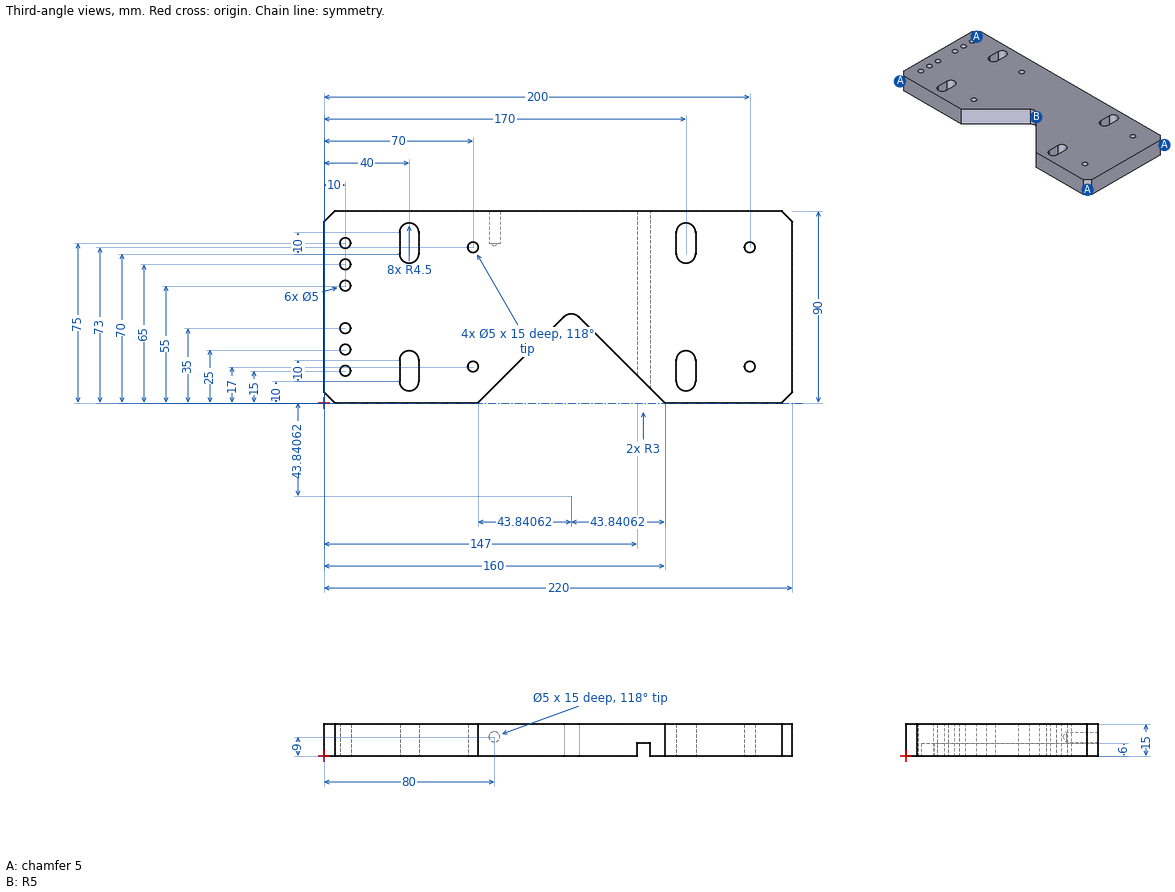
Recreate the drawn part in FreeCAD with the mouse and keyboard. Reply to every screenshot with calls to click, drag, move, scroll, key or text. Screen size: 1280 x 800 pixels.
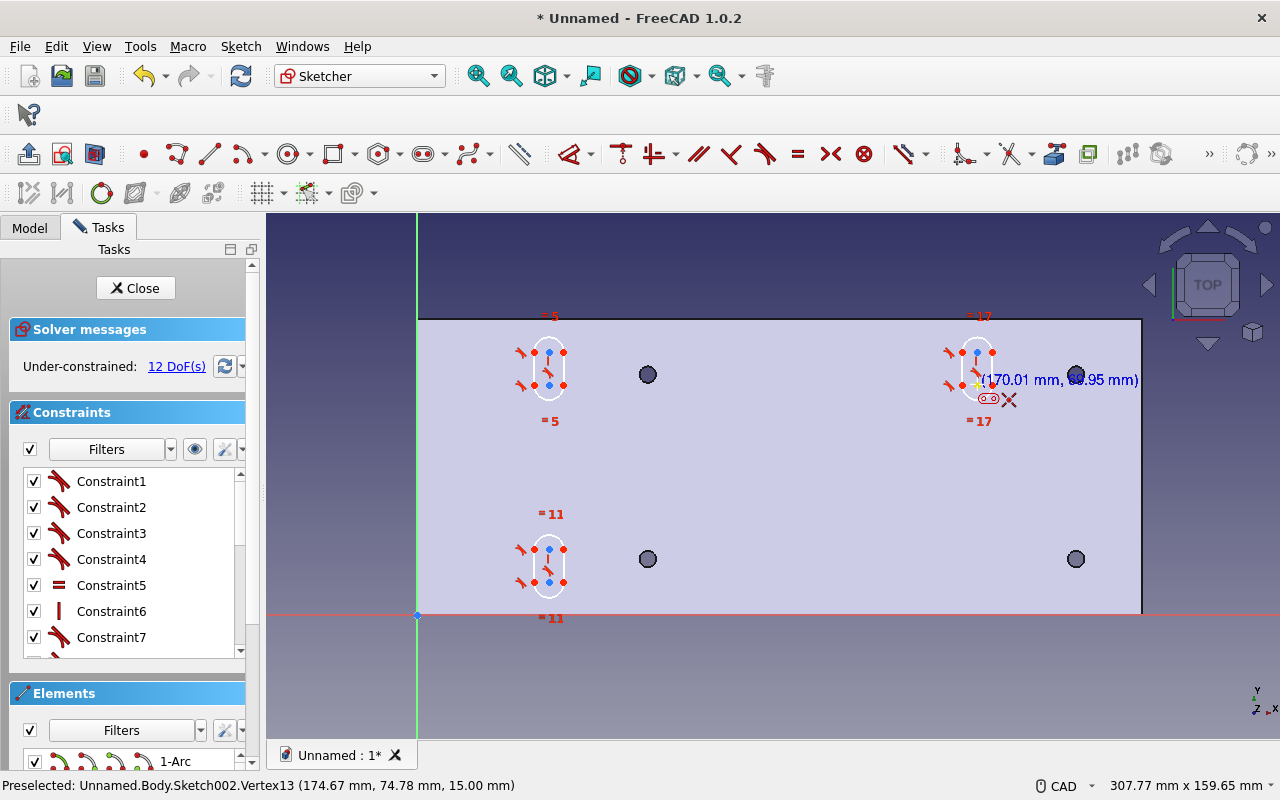
scroll(977, 582, up, 3)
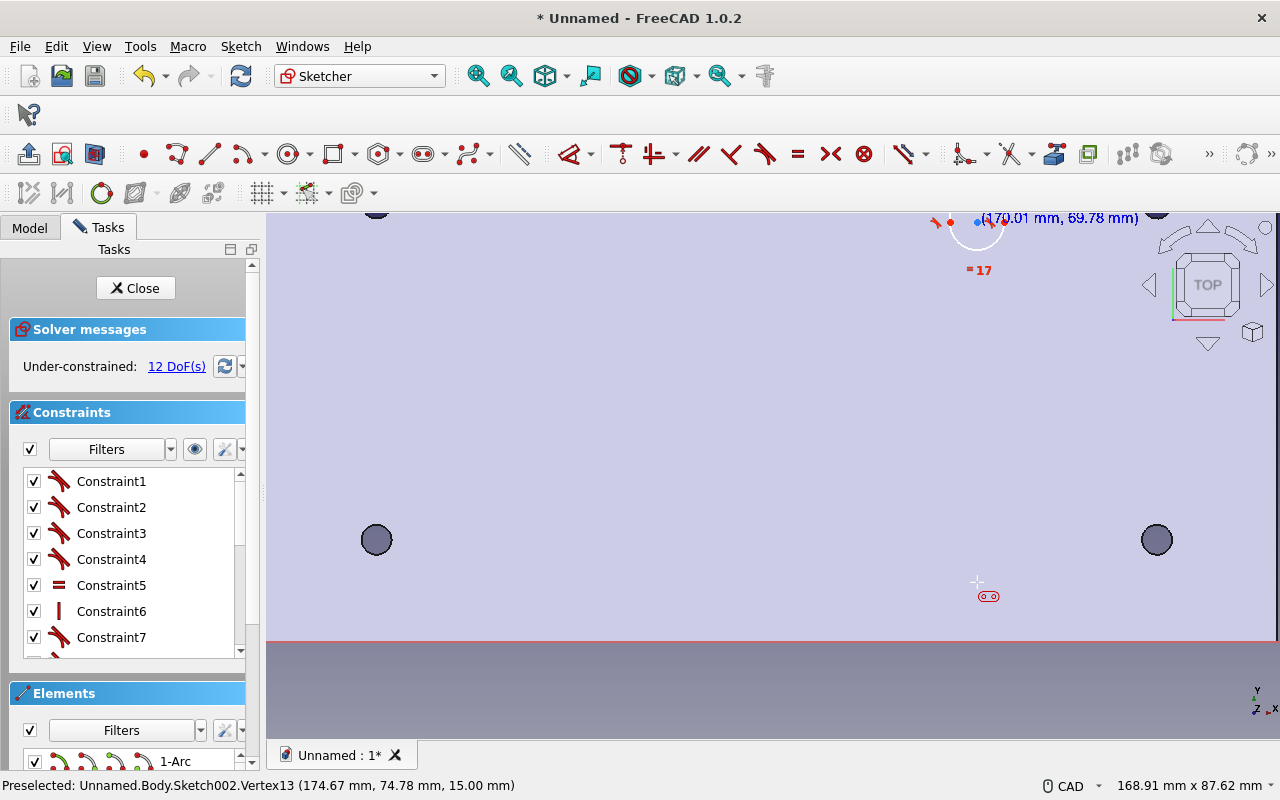
click(977, 582)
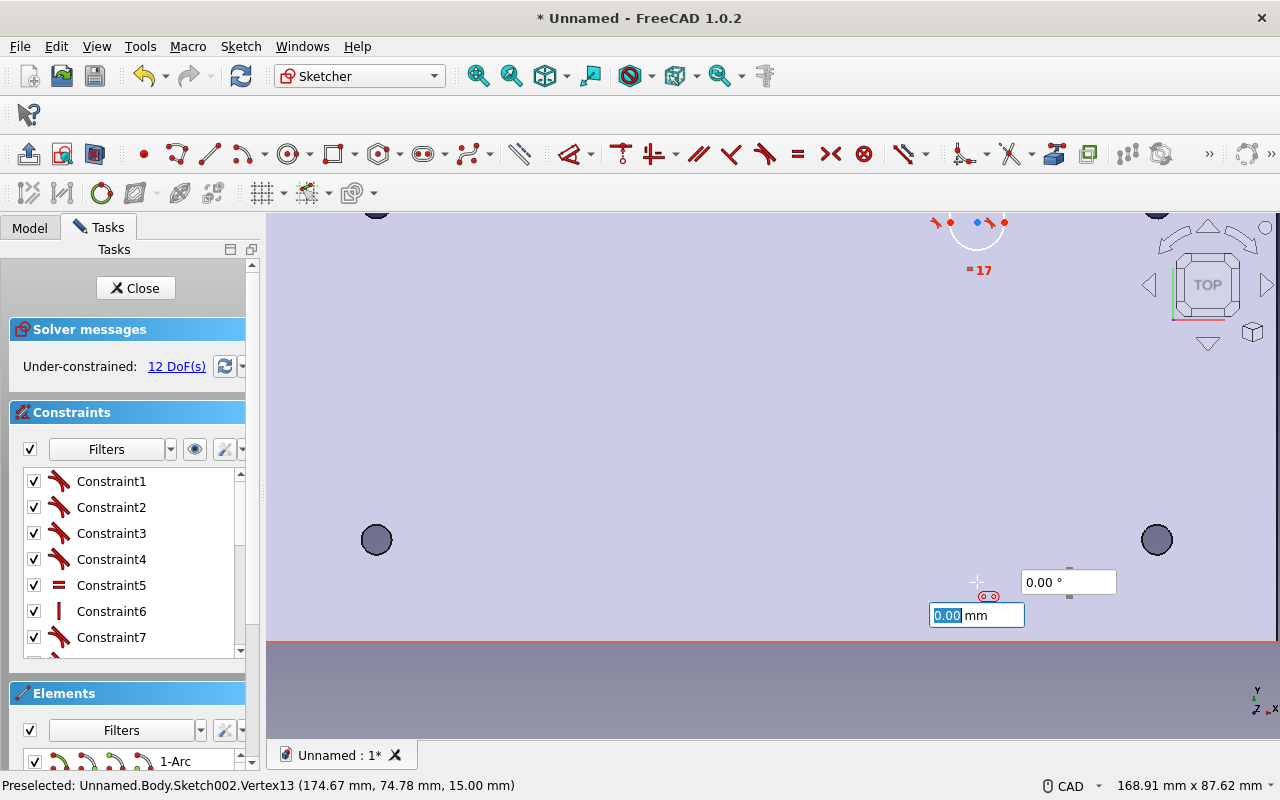
click(977, 522)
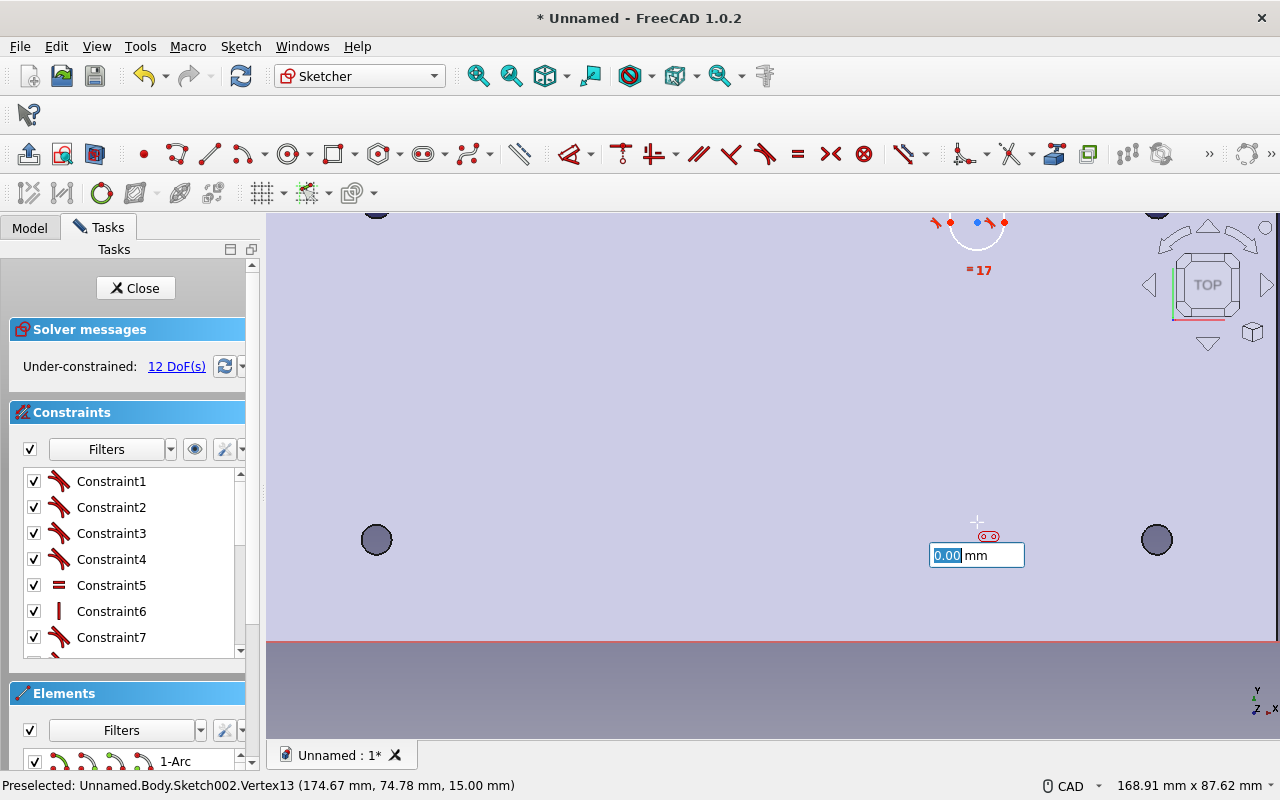
click(1004, 552)
key(Escape)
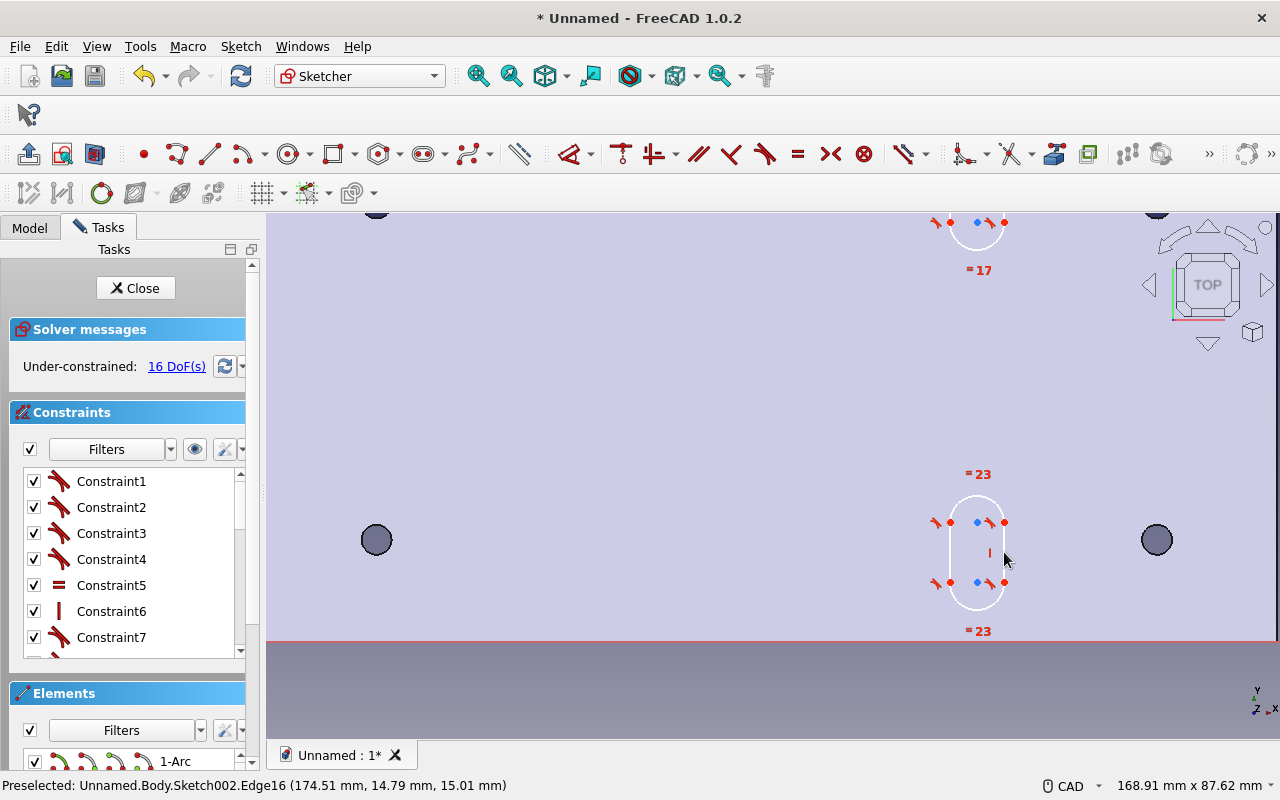
scroll(977, 583, down, 3)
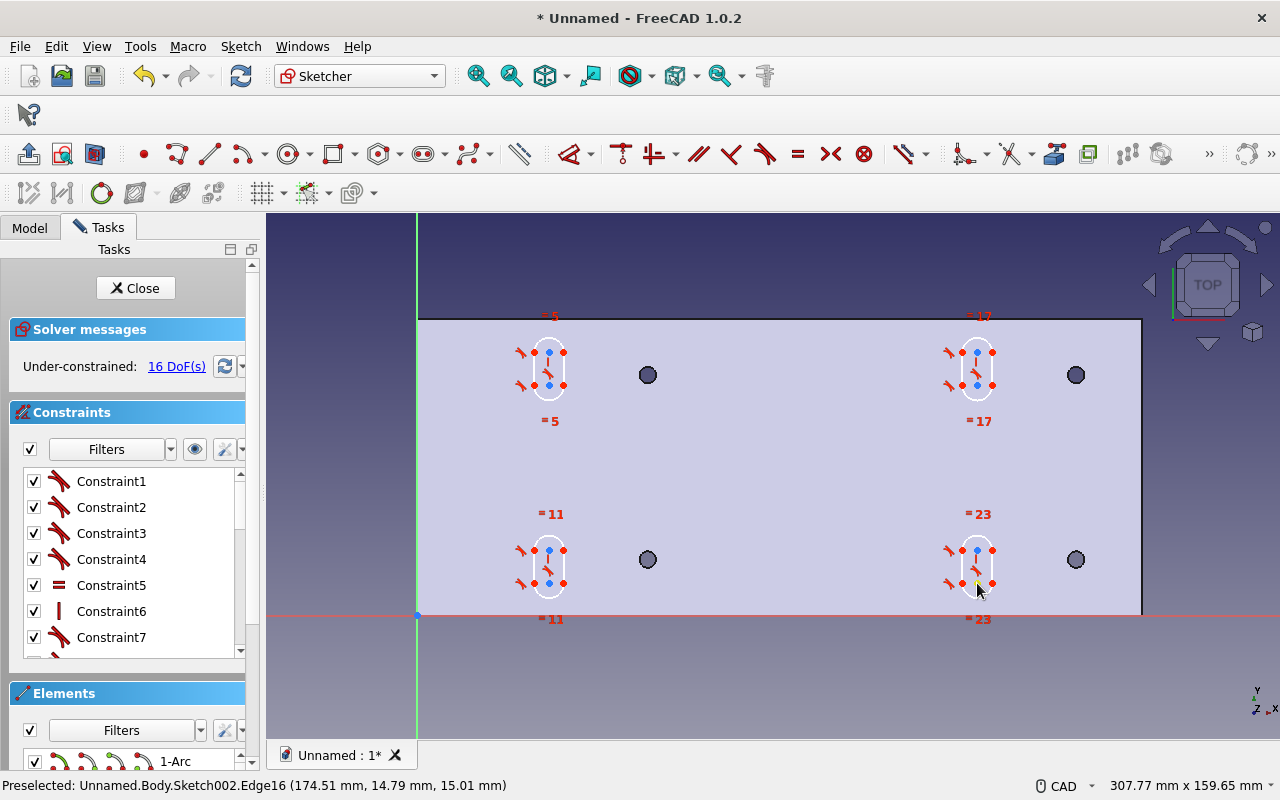
click(540, 398)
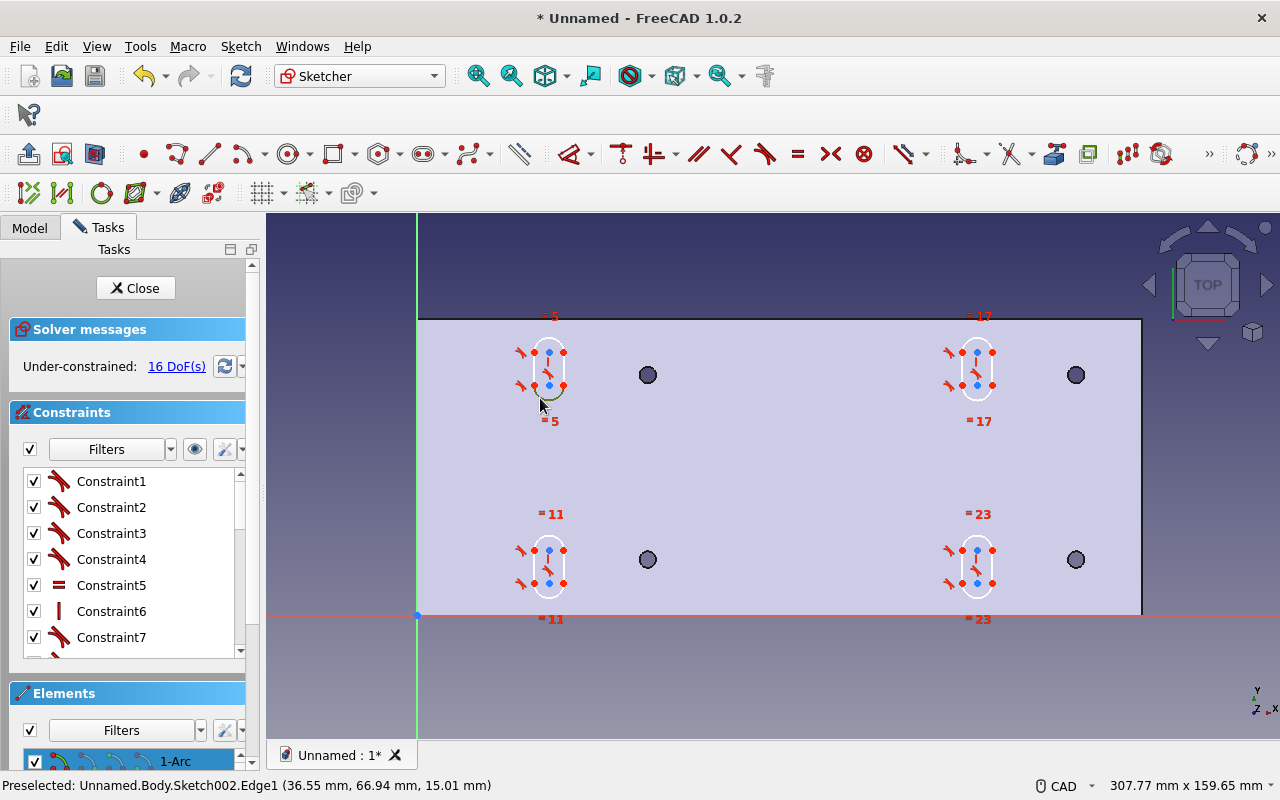
click(540, 595)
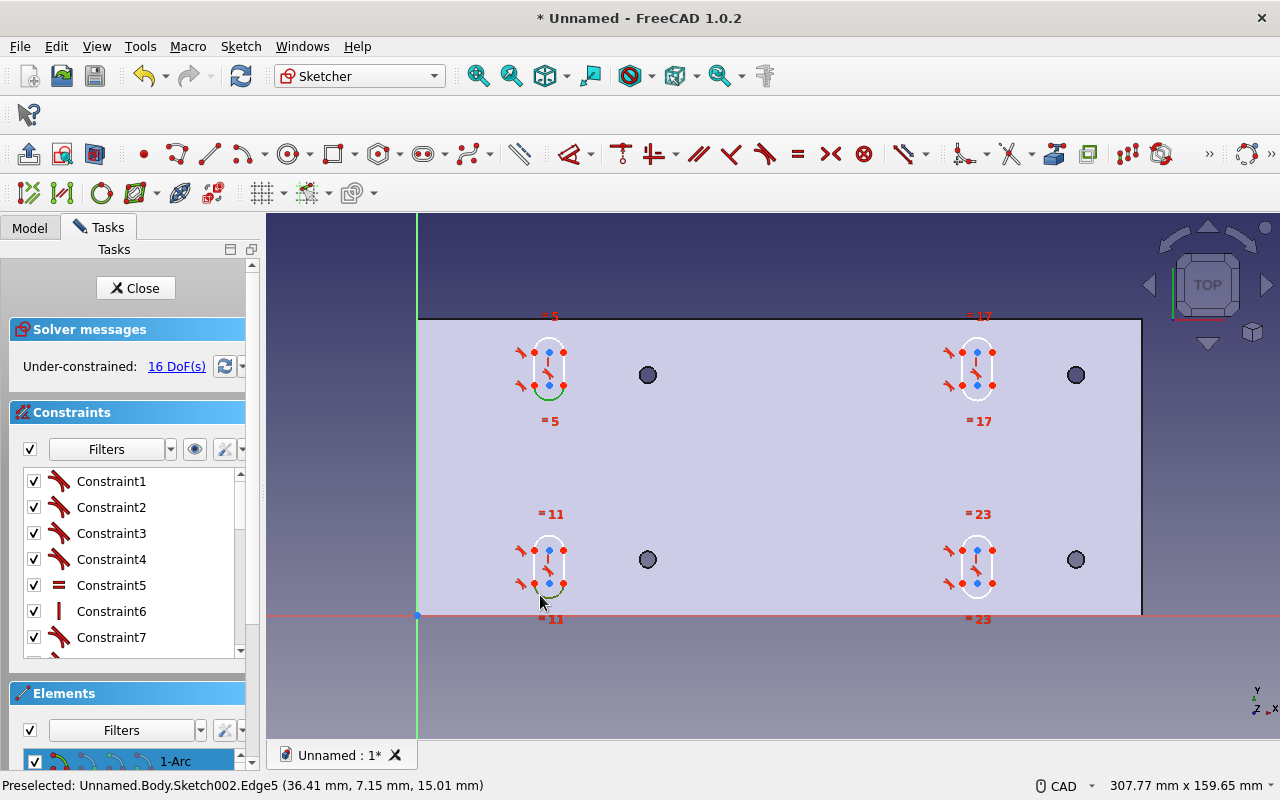
click(969, 398)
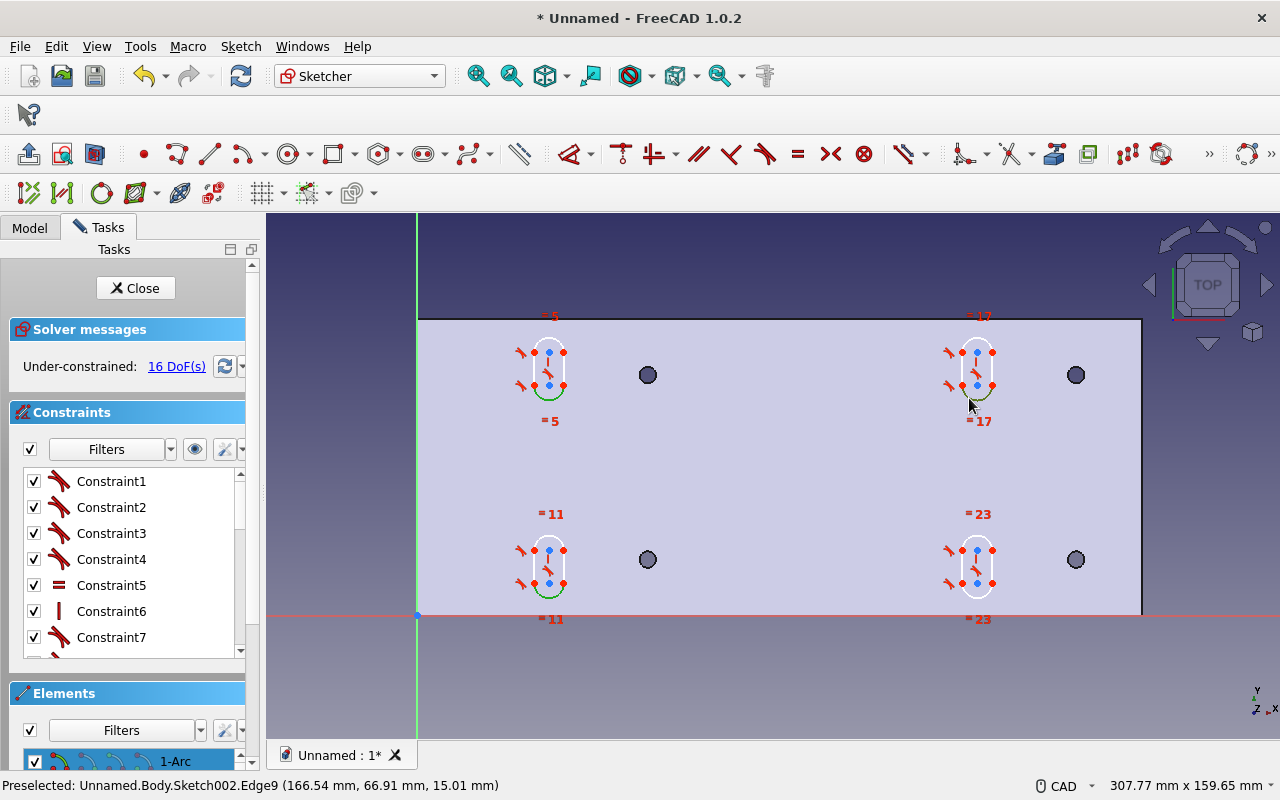
click(969, 595)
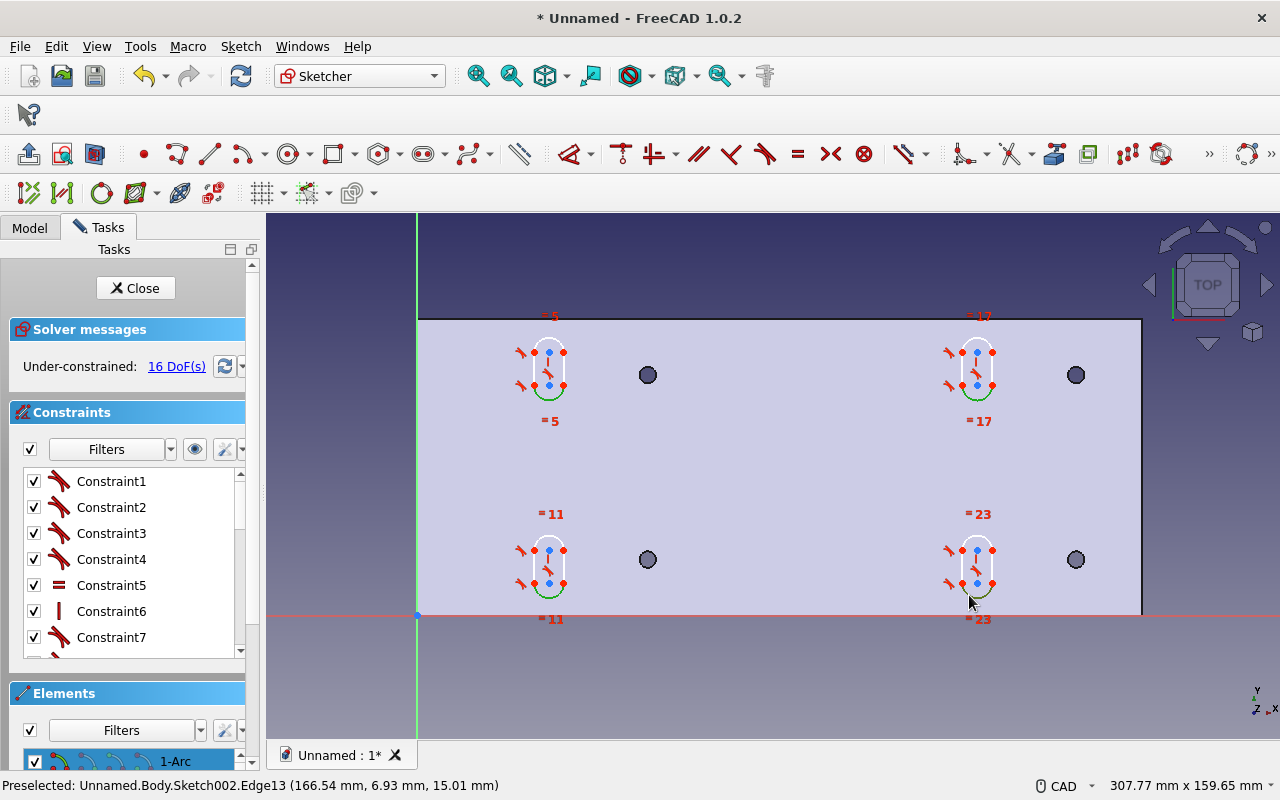
click(798, 154)